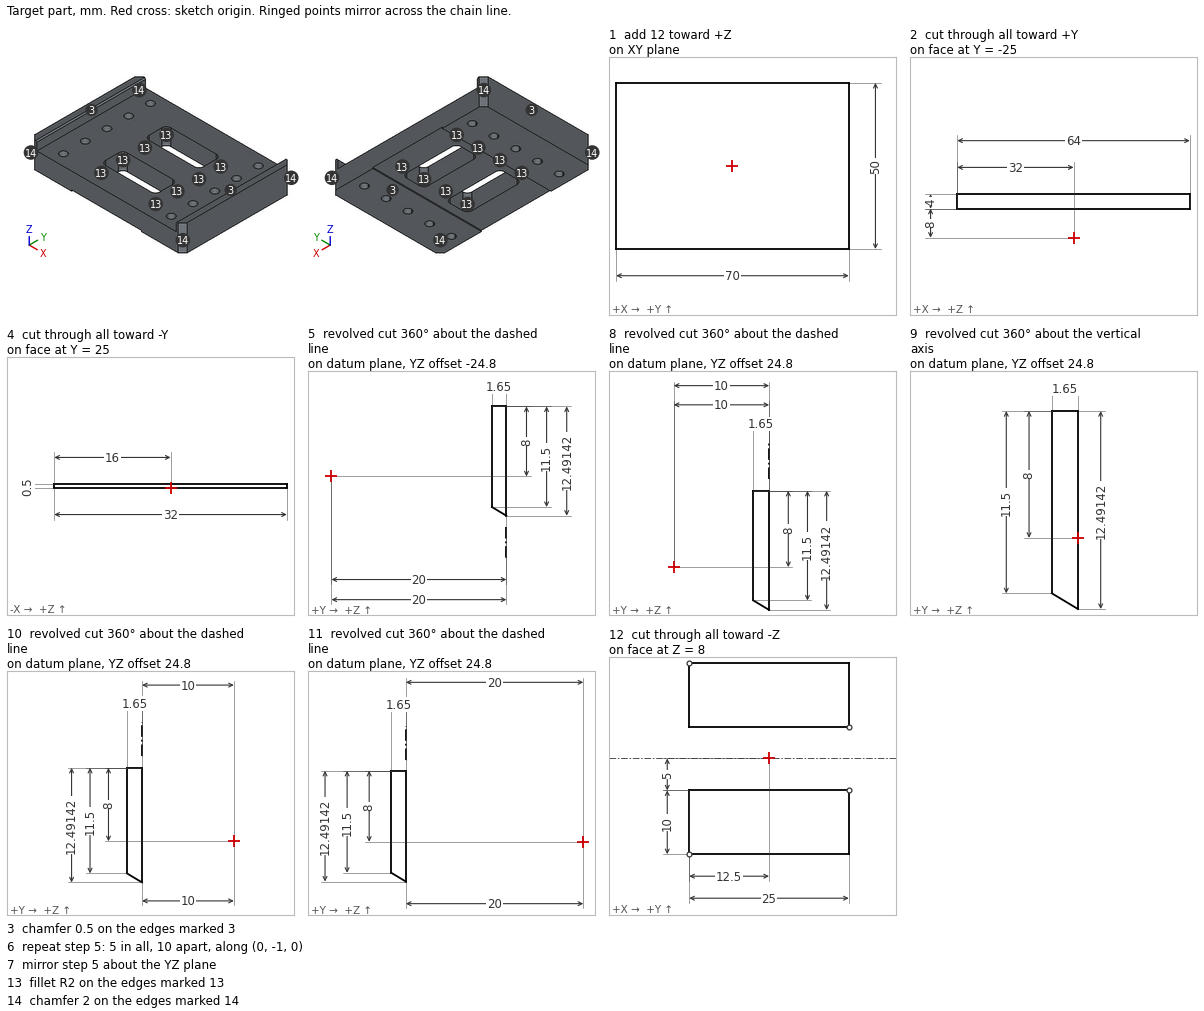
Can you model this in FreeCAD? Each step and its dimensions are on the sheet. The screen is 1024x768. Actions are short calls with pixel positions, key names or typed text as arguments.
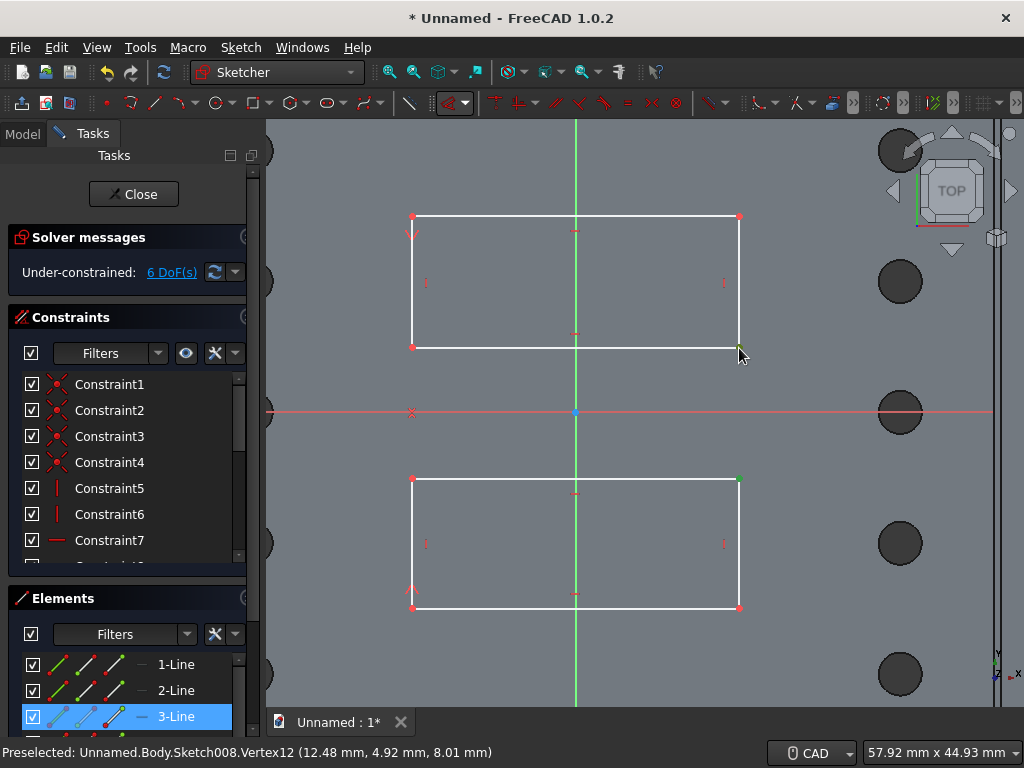
click(334, 412)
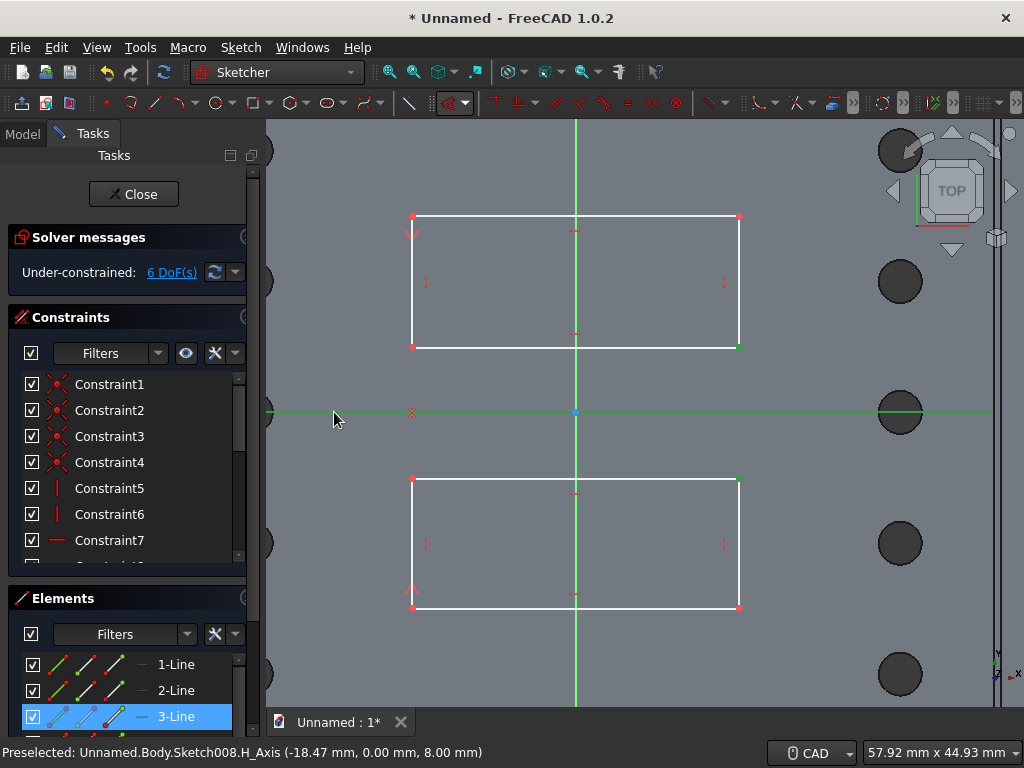
key(s)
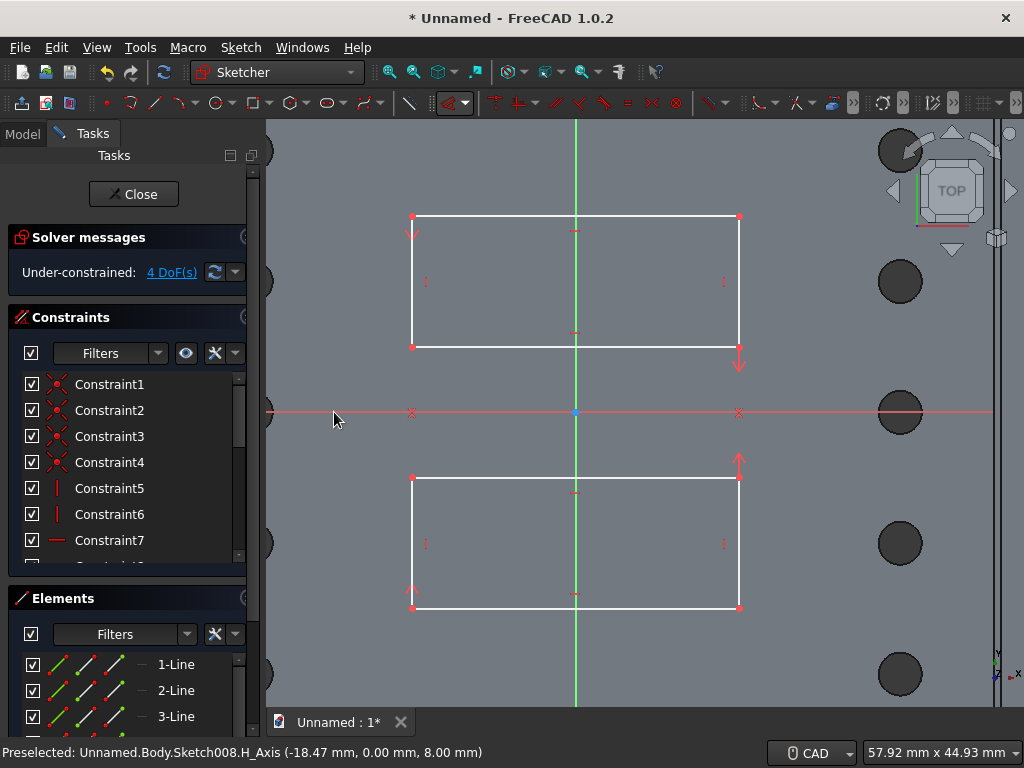
click(412, 517)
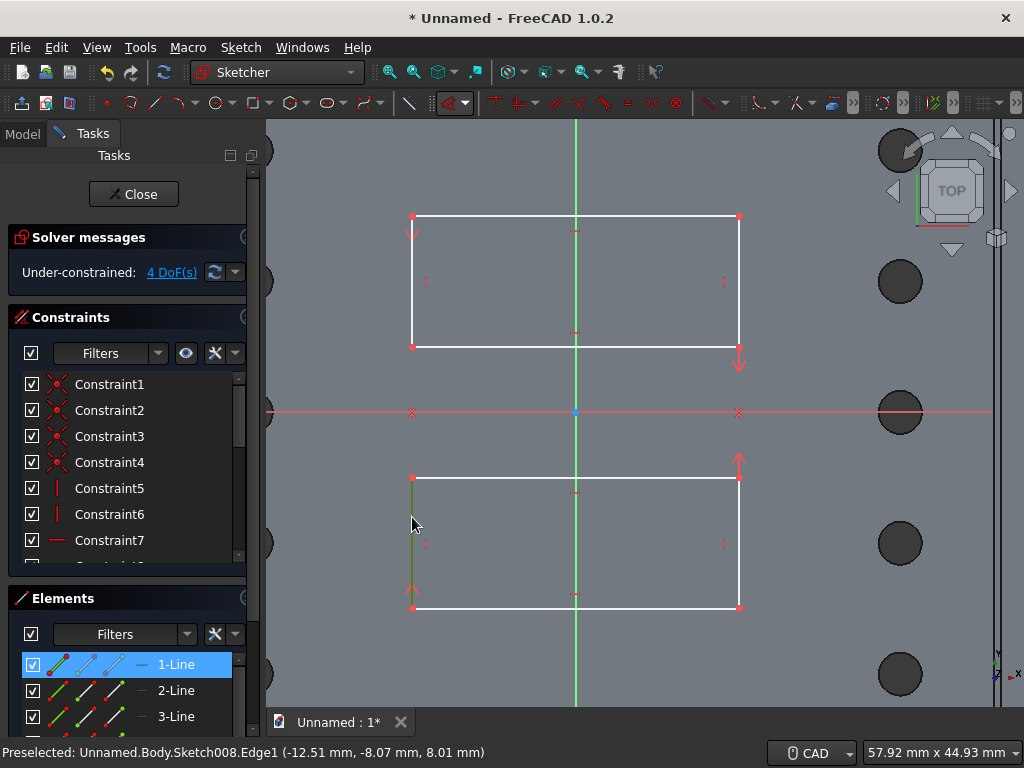
key(i)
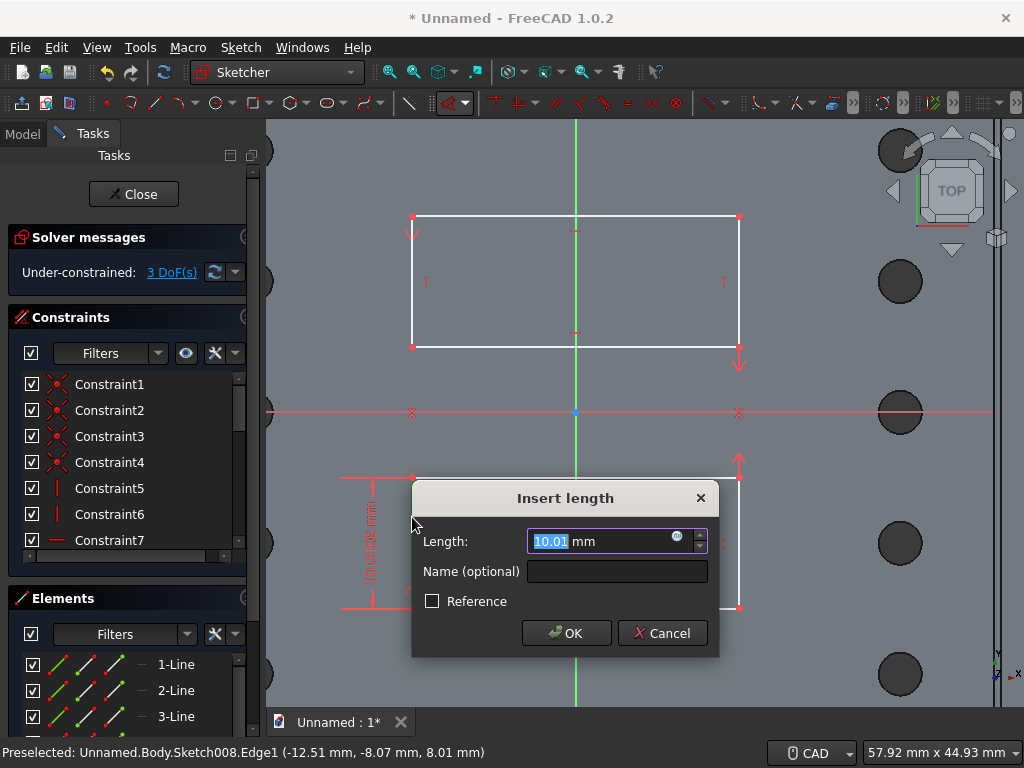
text(10)
key(Return)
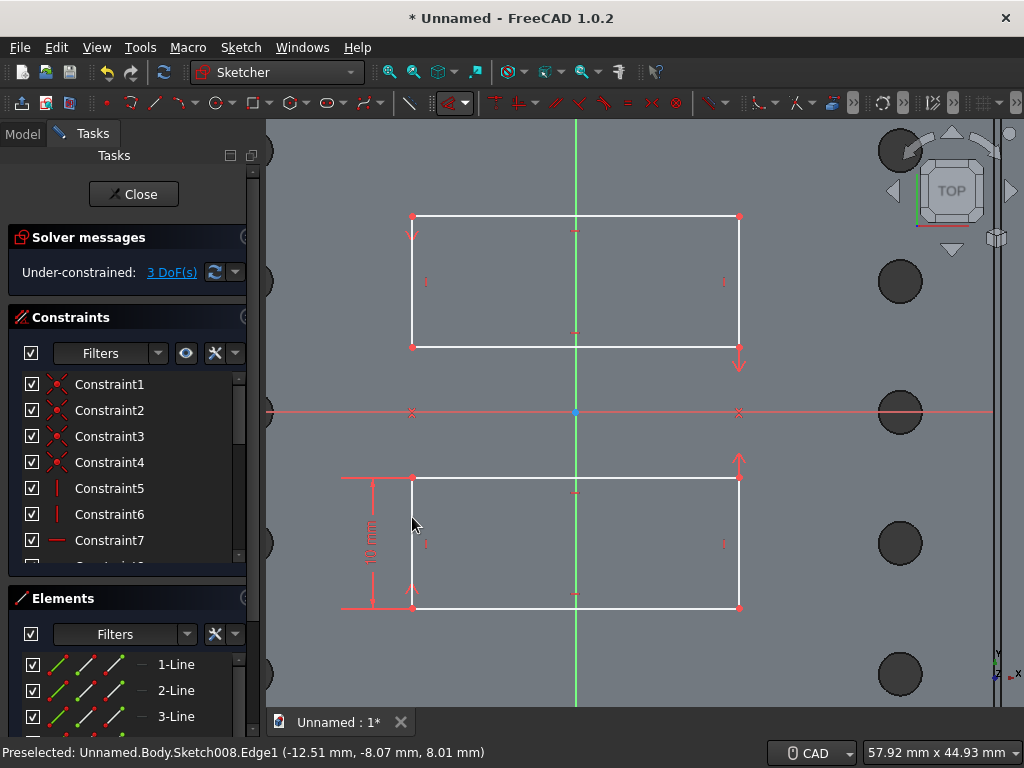
click(510, 609)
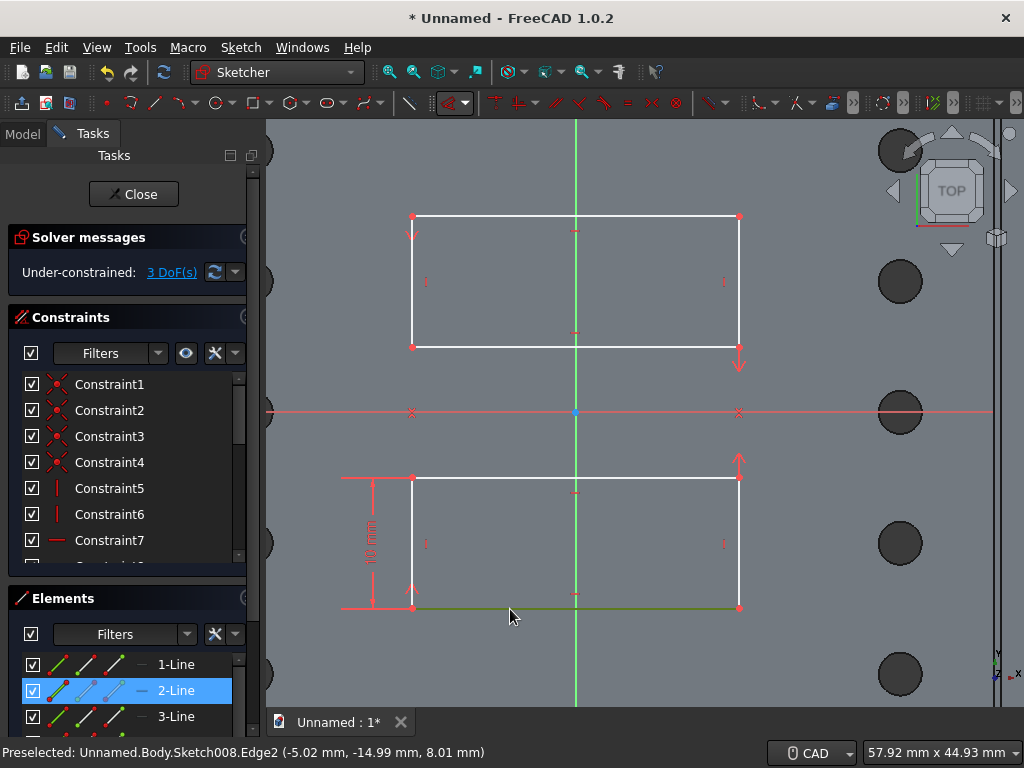
click(468, 104)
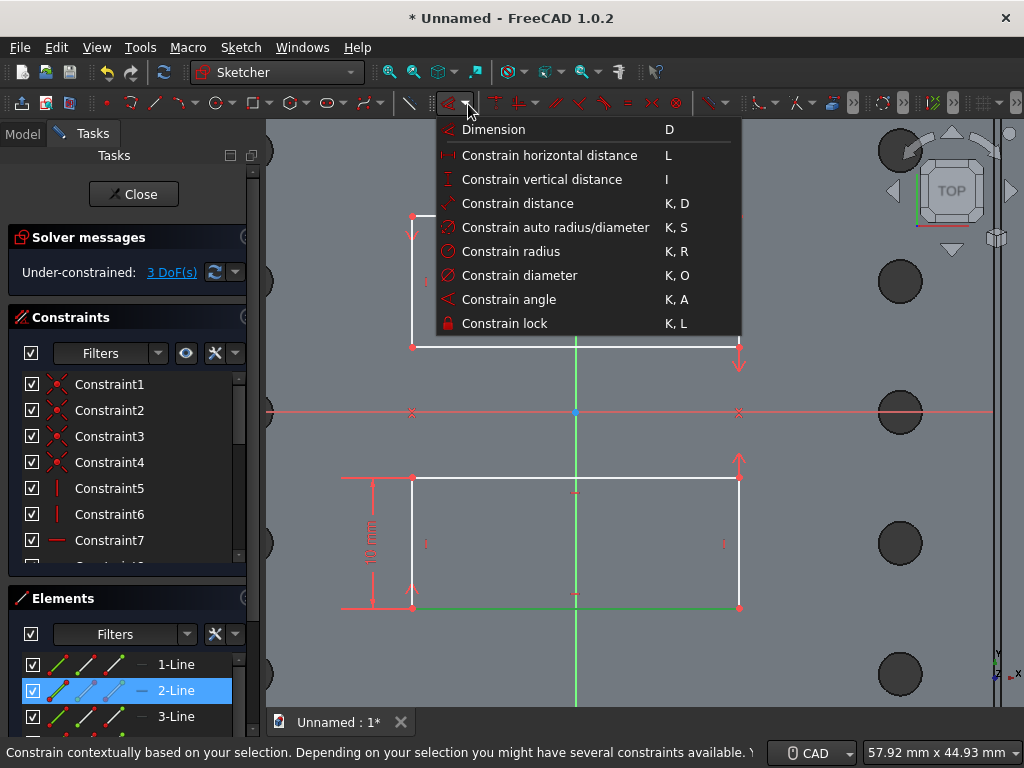
click(589, 155)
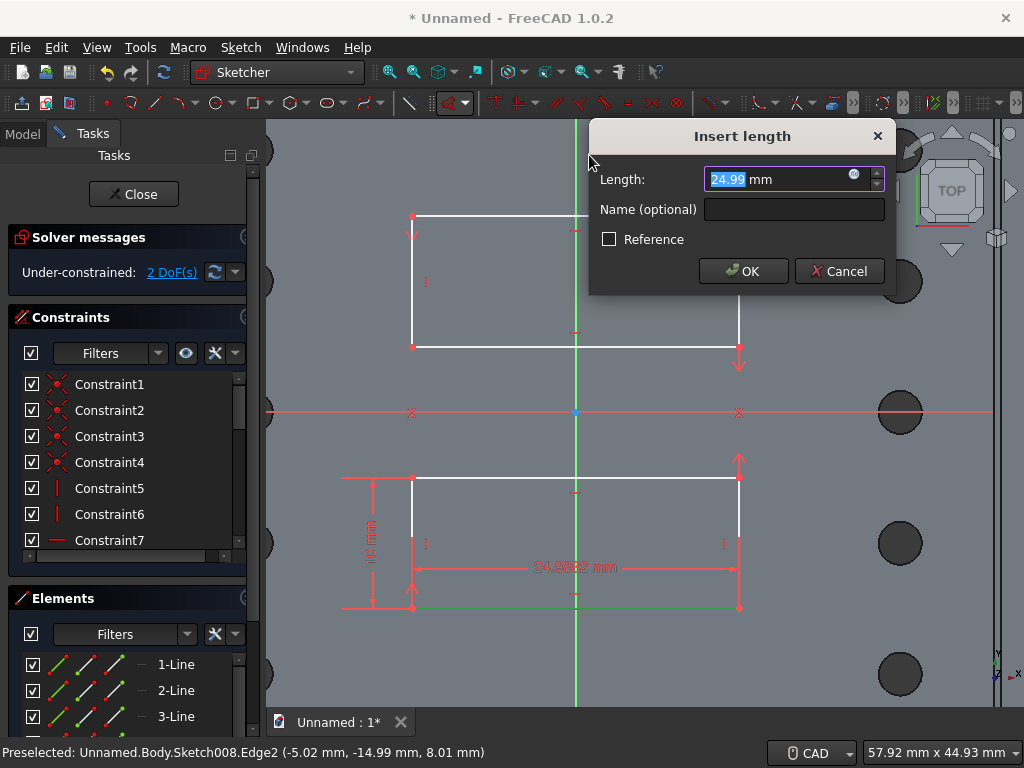
text(25)
key(Return)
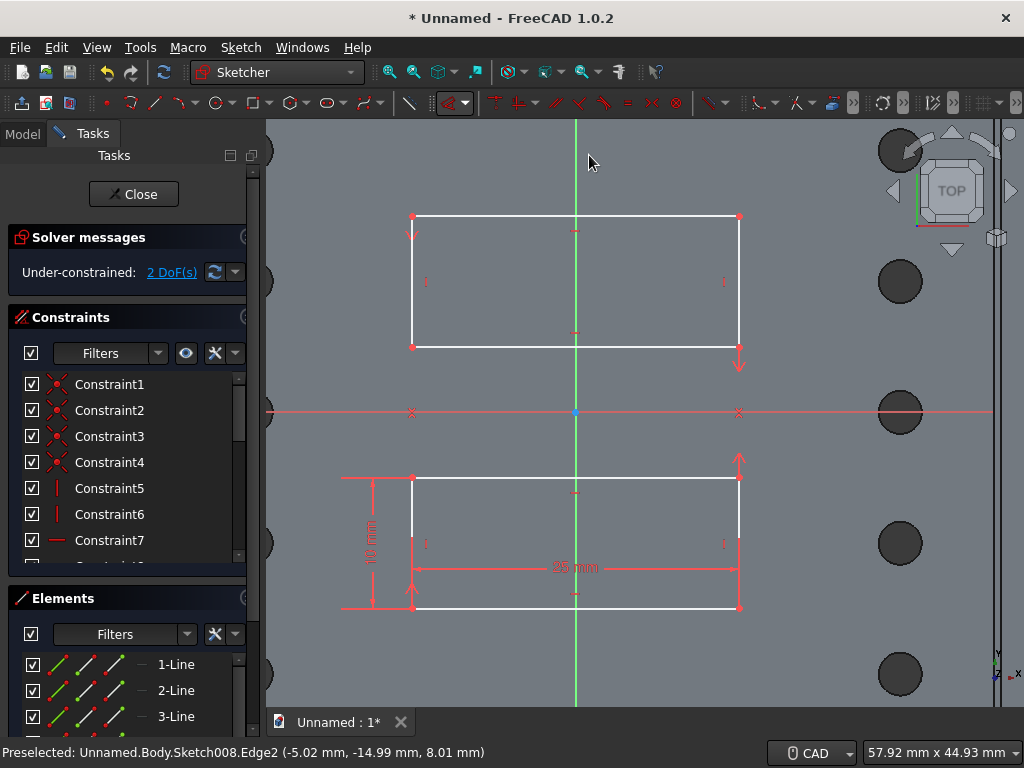
click(412, 478)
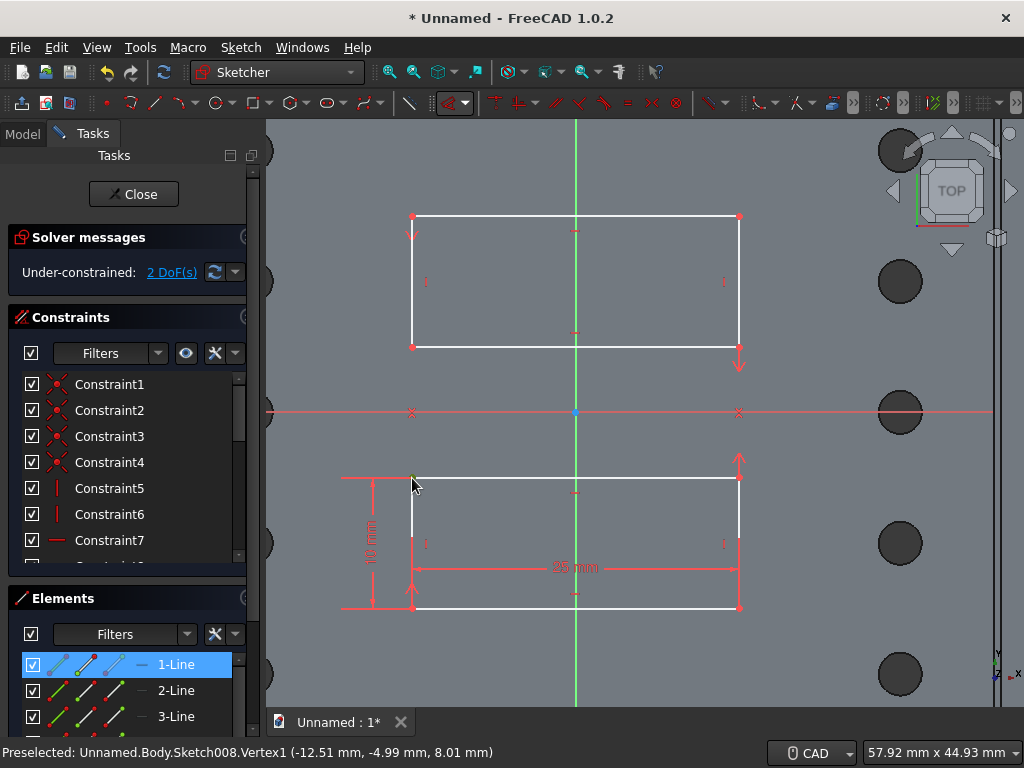
key(i)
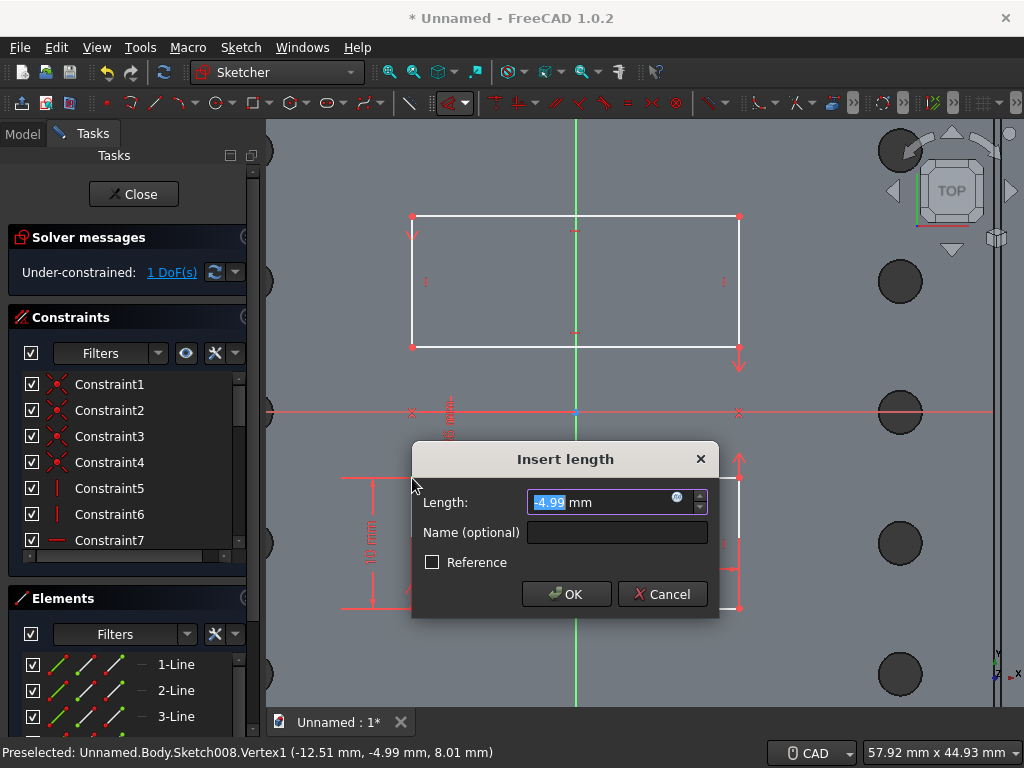
text(-5)
key(Return)